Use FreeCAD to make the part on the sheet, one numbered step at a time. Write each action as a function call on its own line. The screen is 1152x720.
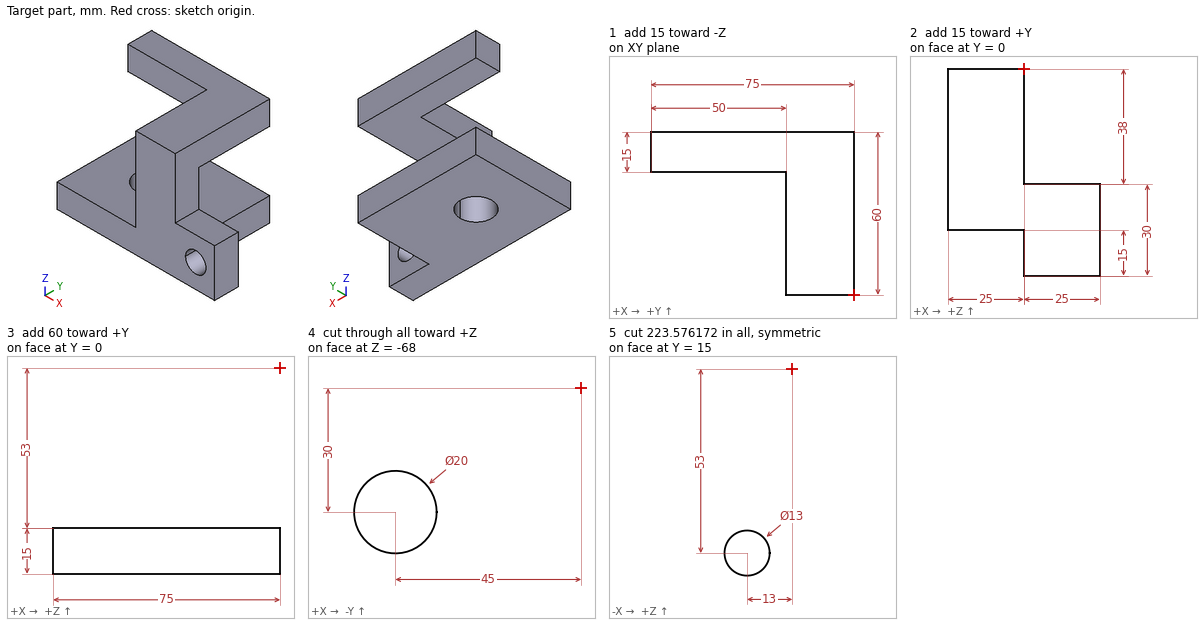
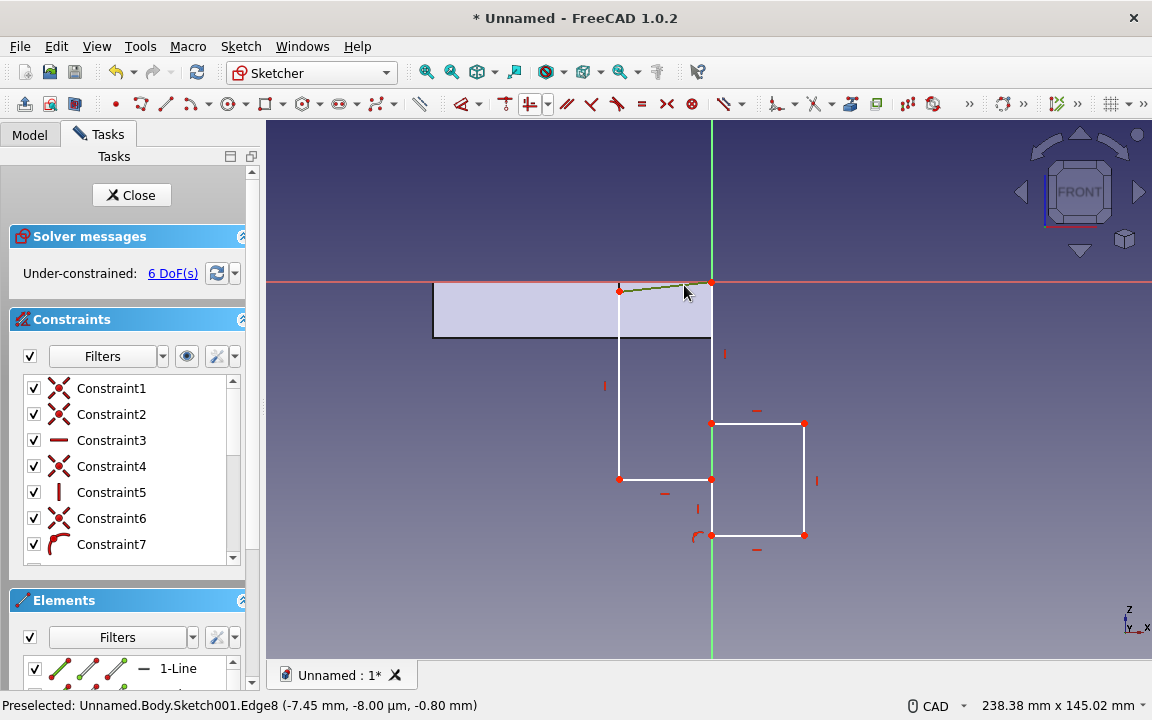
key(h)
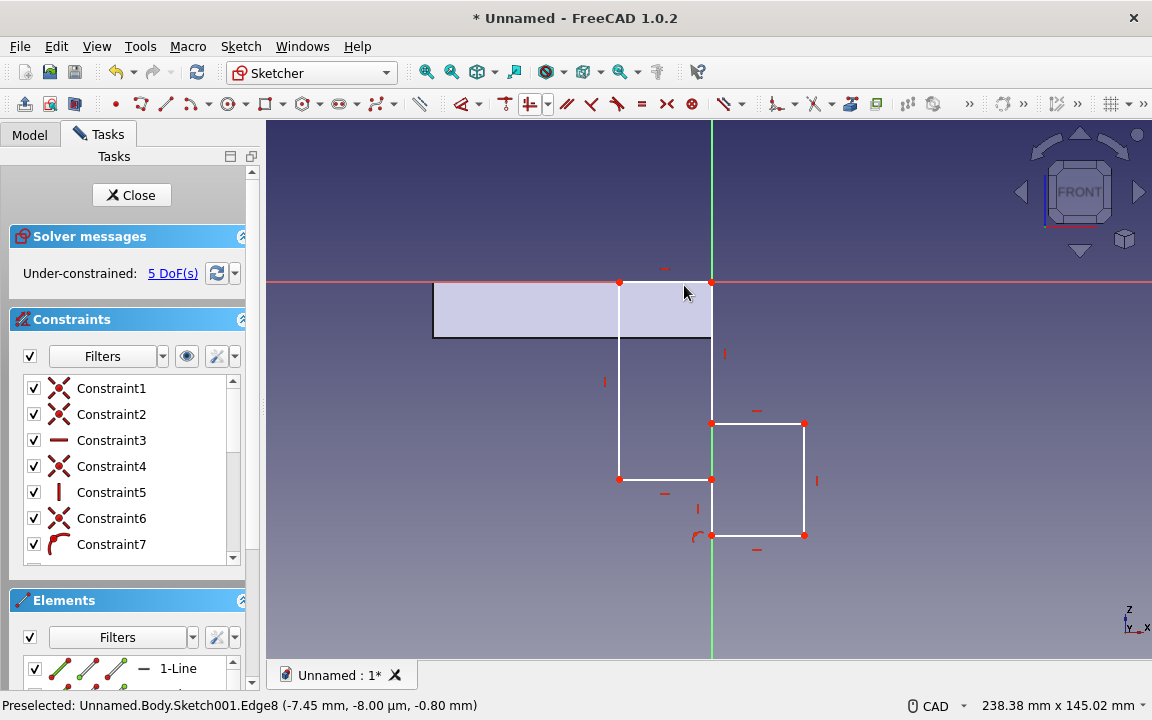
key(d)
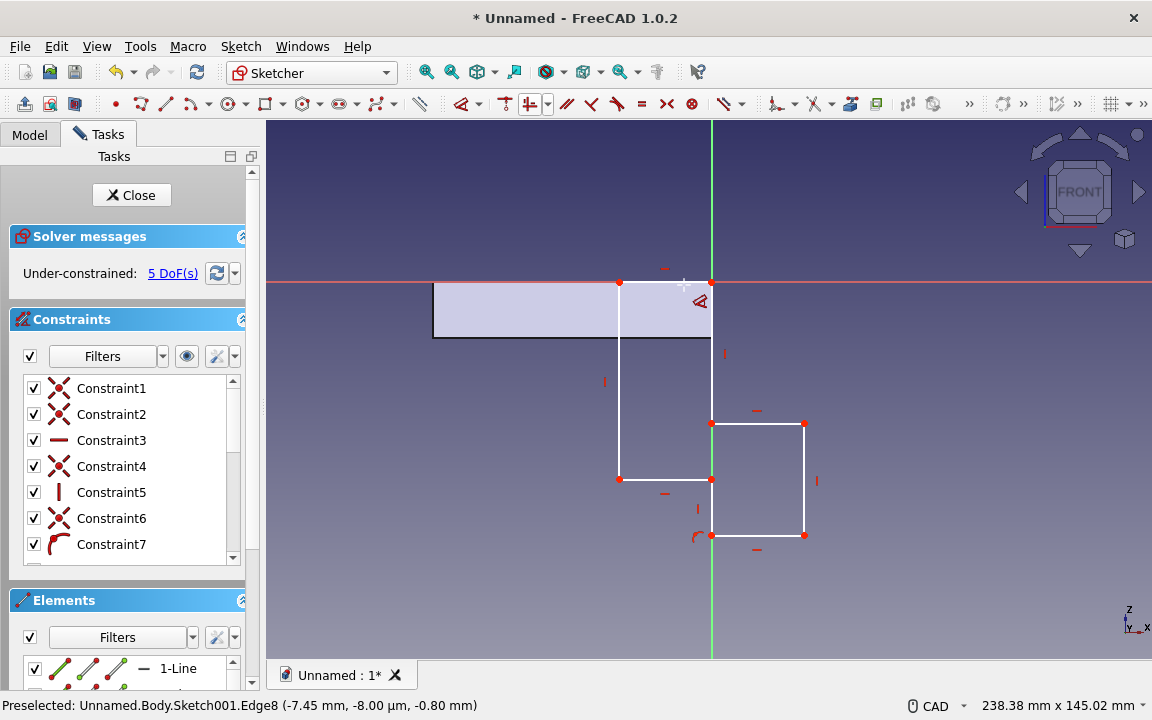
click(712, 325)
click(746, 353)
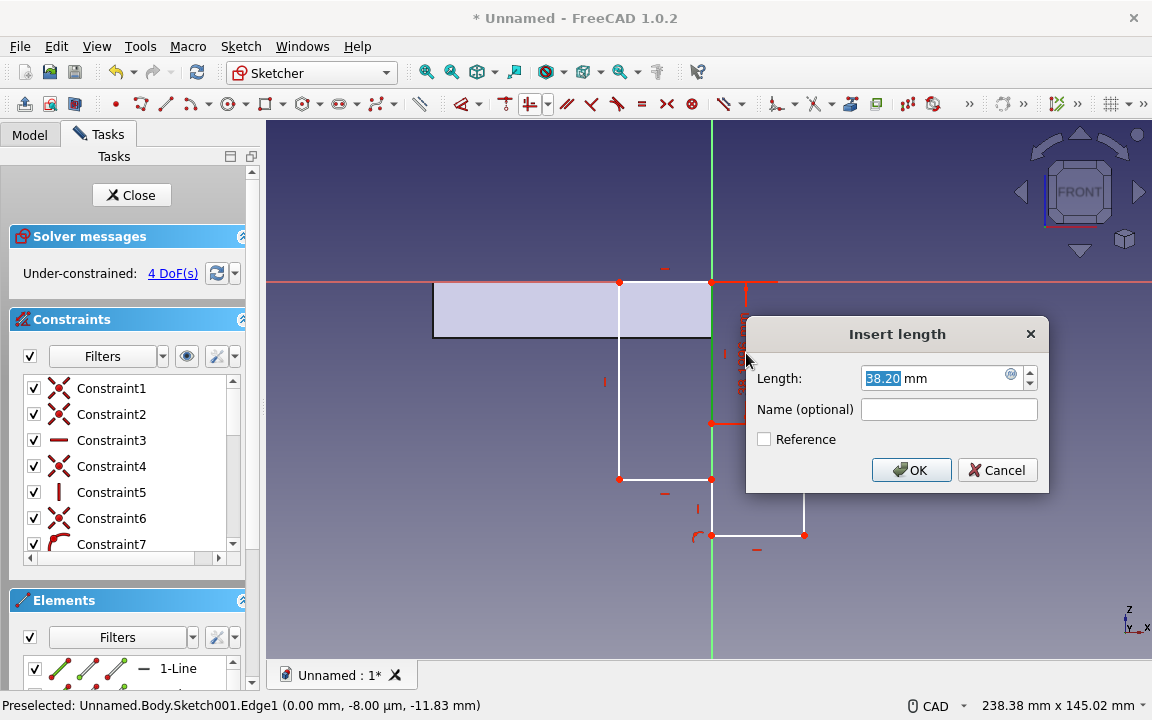
text(38)
key(Return)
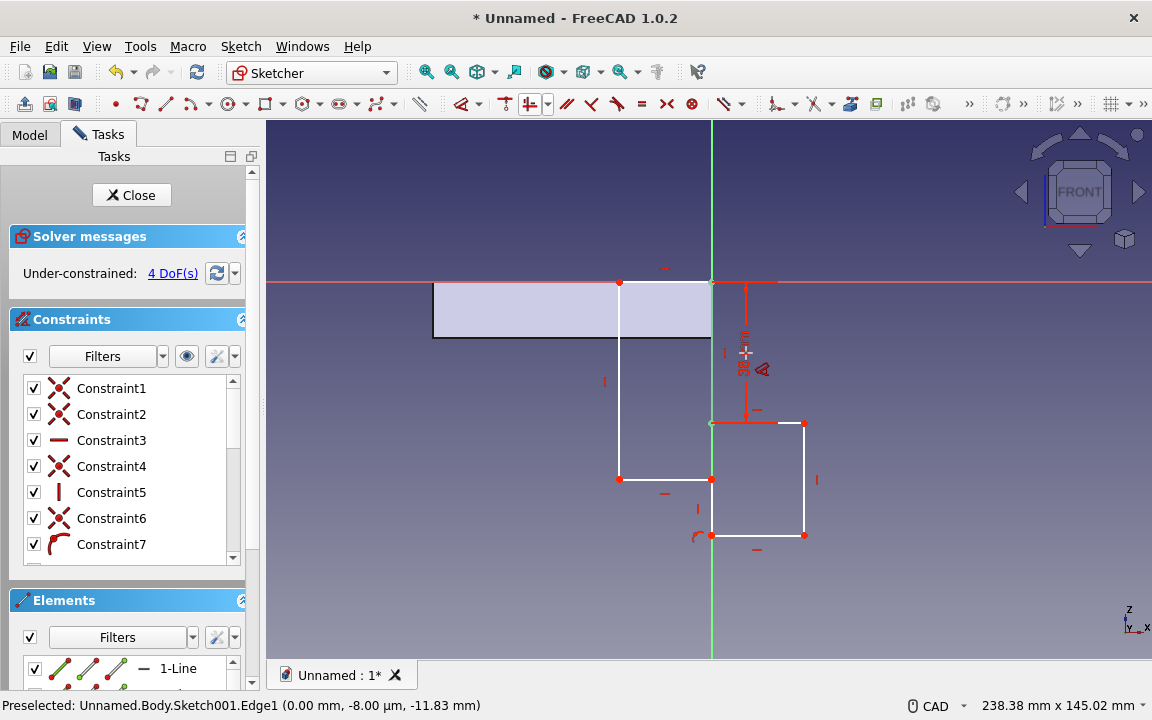
click(739, 423)
click(758, 457)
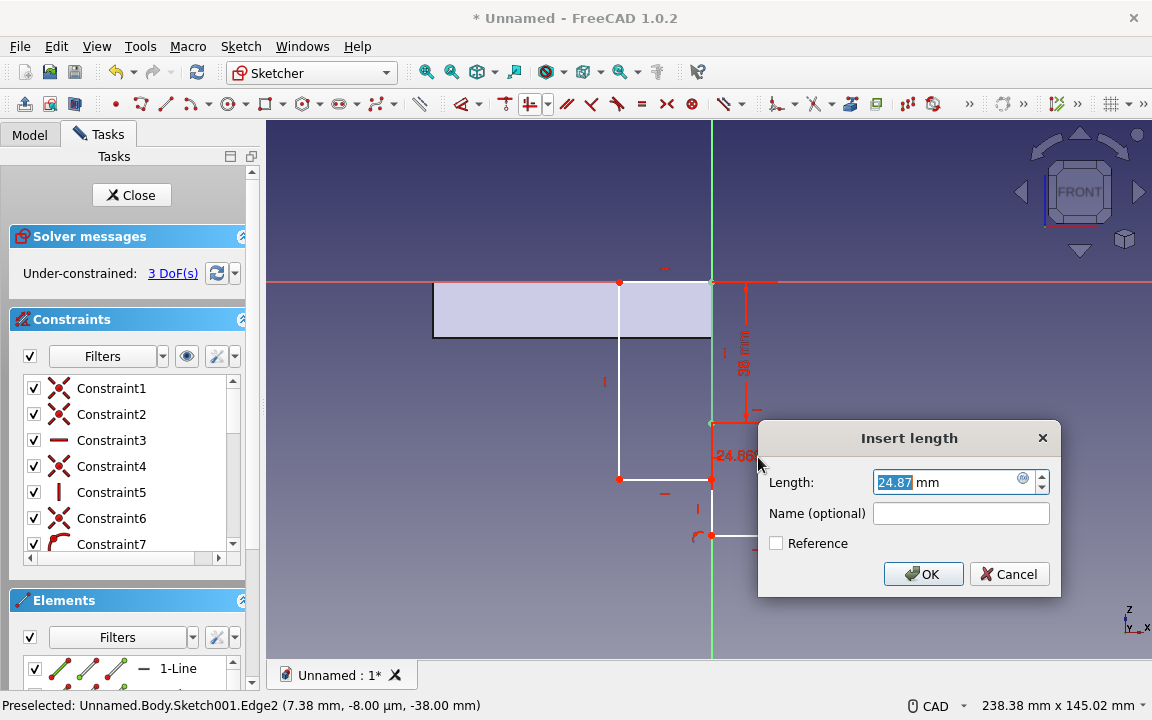
text(25)
key(Return)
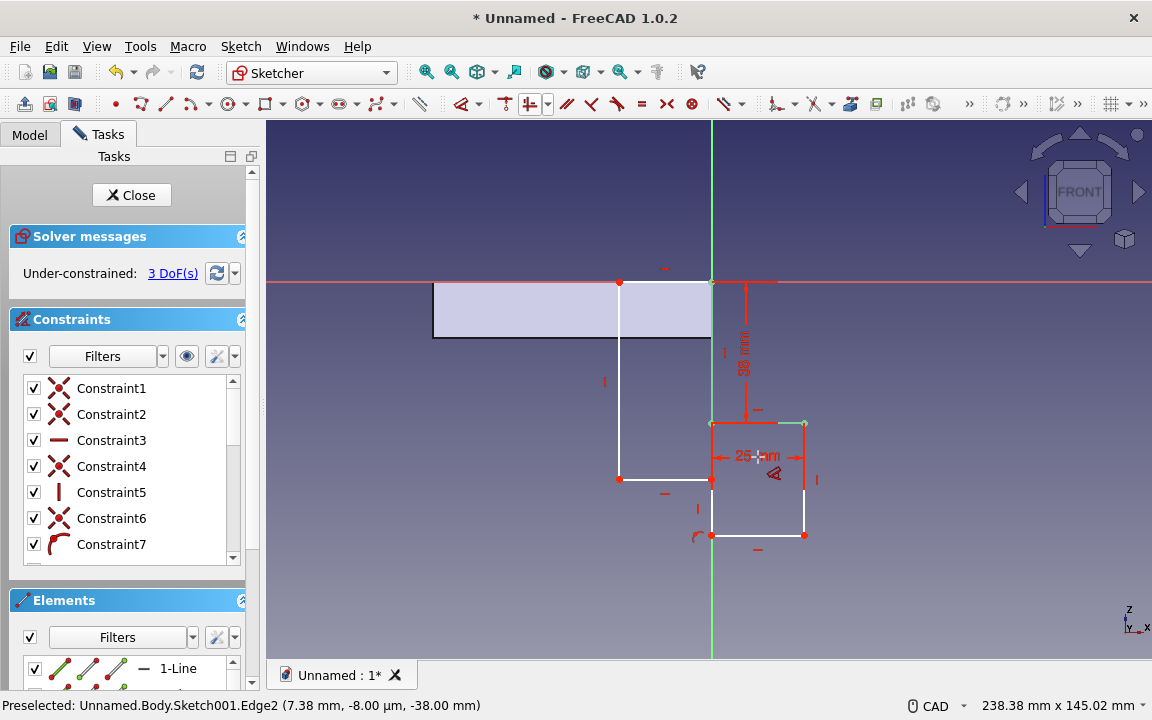
click(804, 457)
click(838, 480)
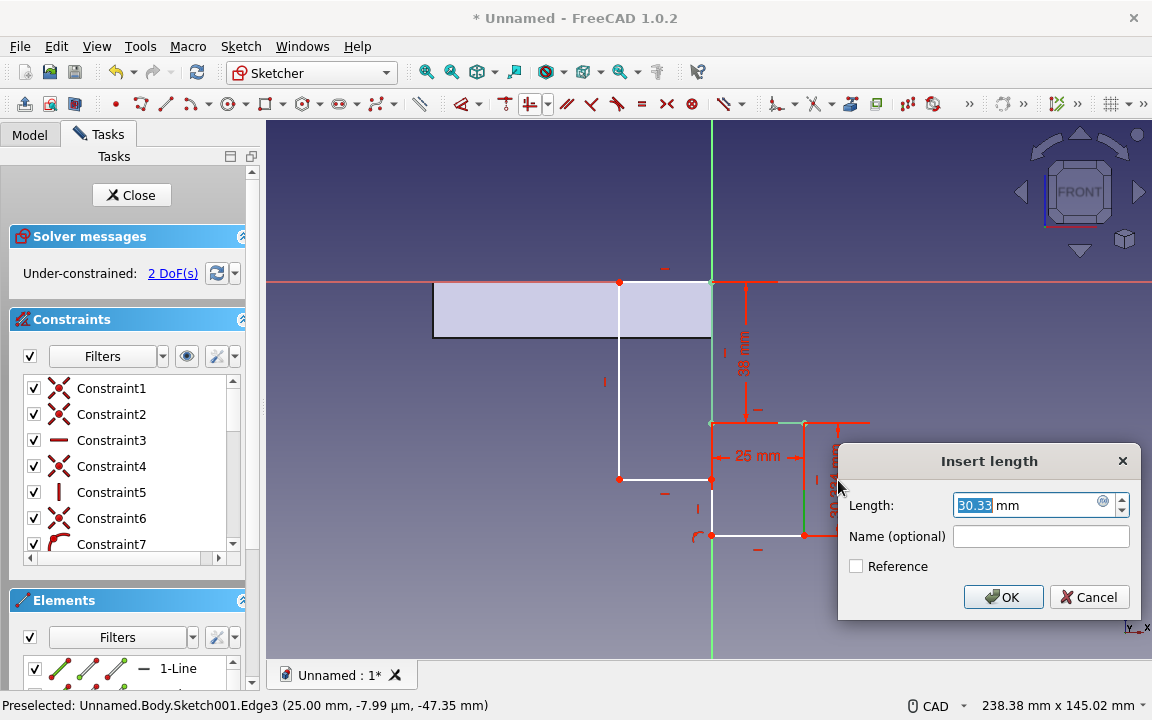
text(30)
key(Return)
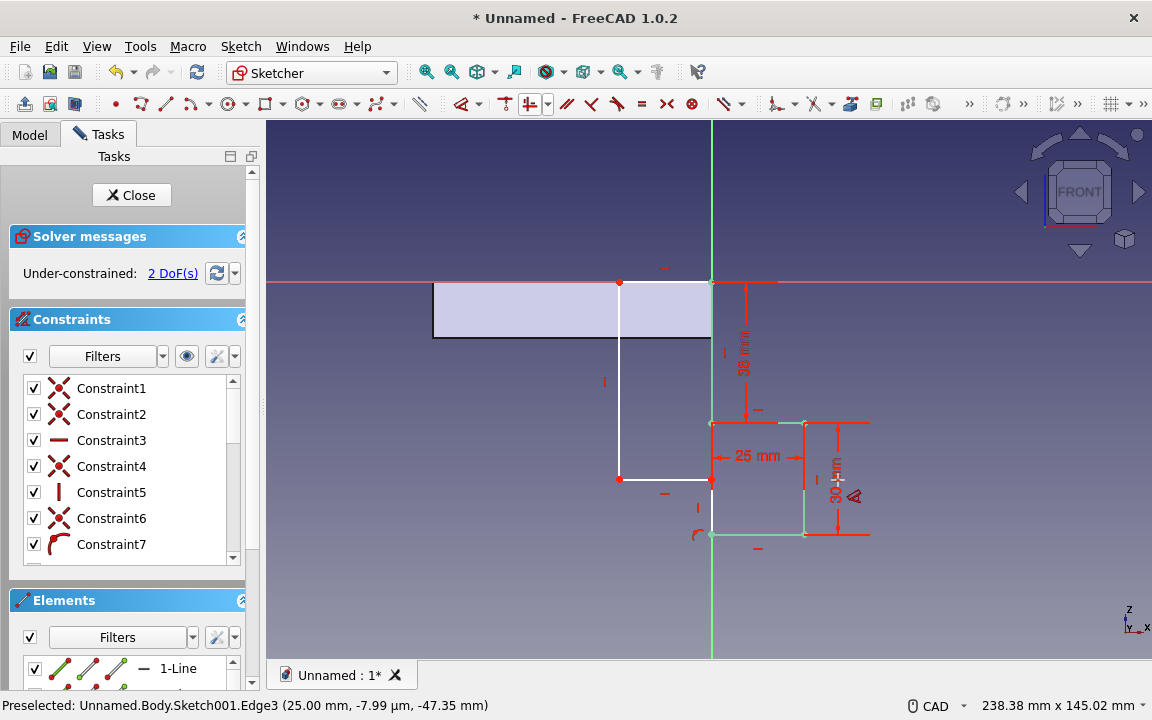
click(712, 518)
click(746, 507)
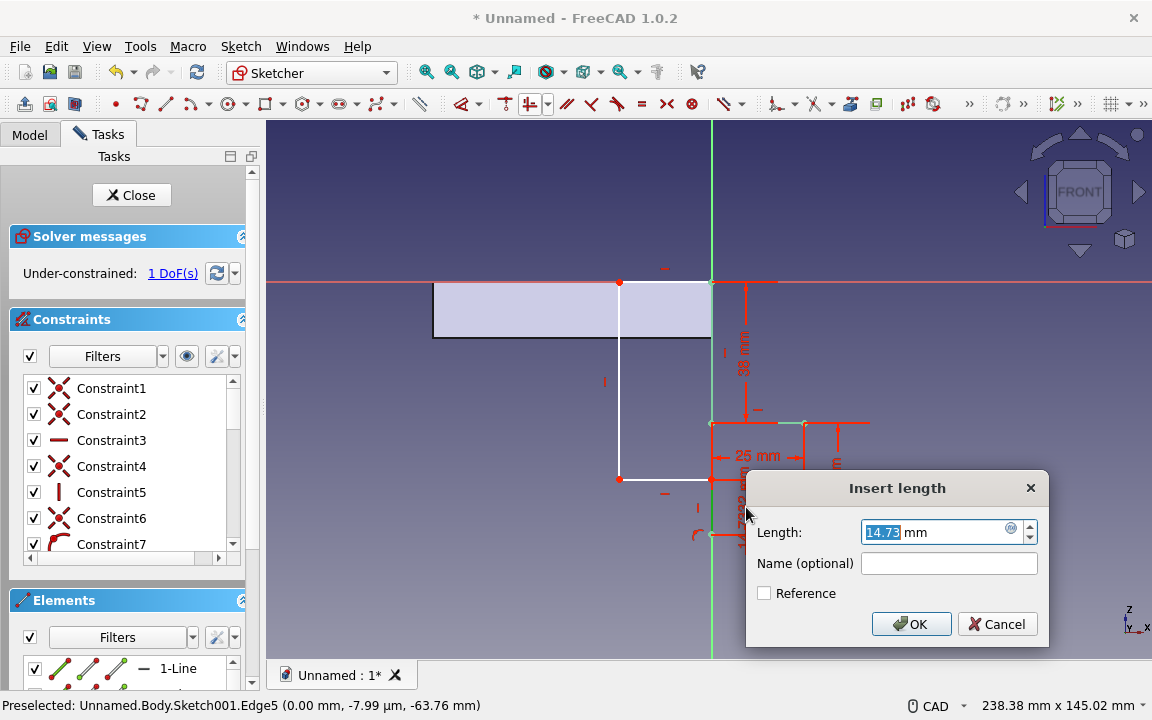
text(15)
key(Return)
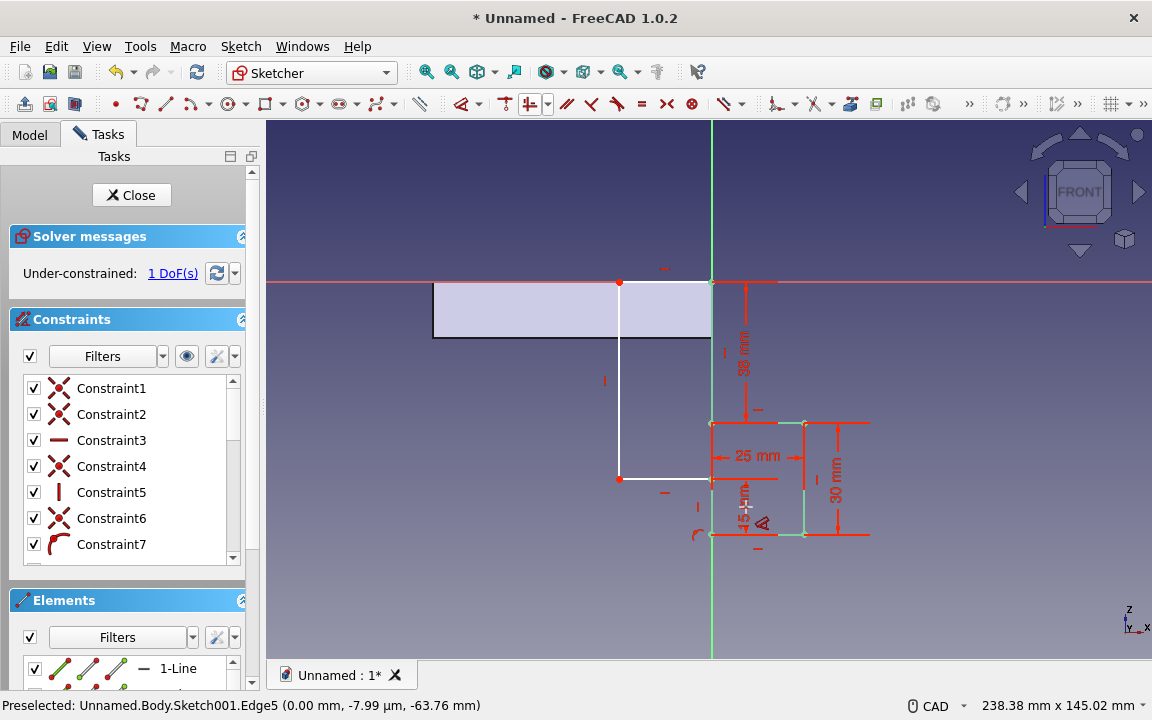
click(684, 479)
click(665, 513)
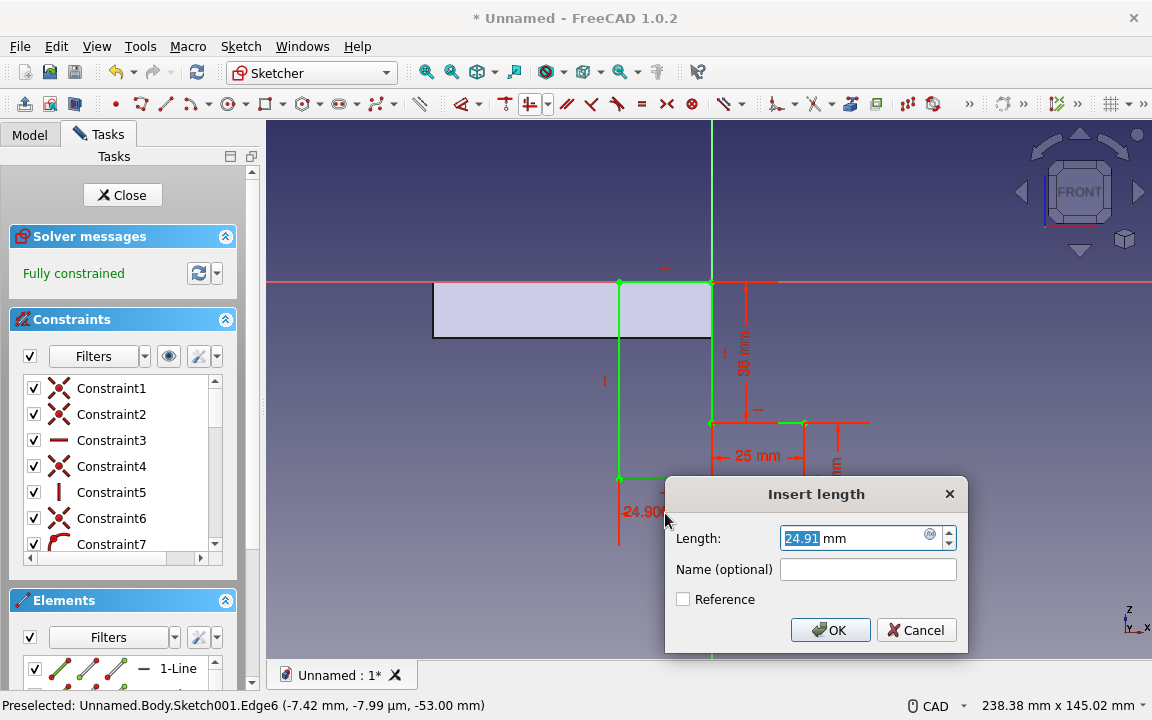
text(25)
key(Return)
key(Escape)